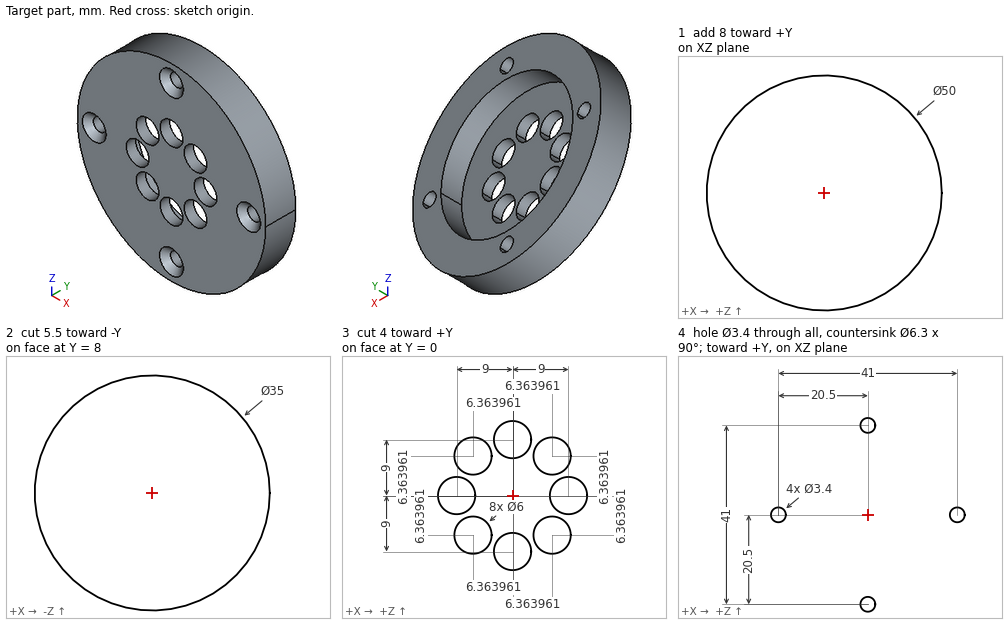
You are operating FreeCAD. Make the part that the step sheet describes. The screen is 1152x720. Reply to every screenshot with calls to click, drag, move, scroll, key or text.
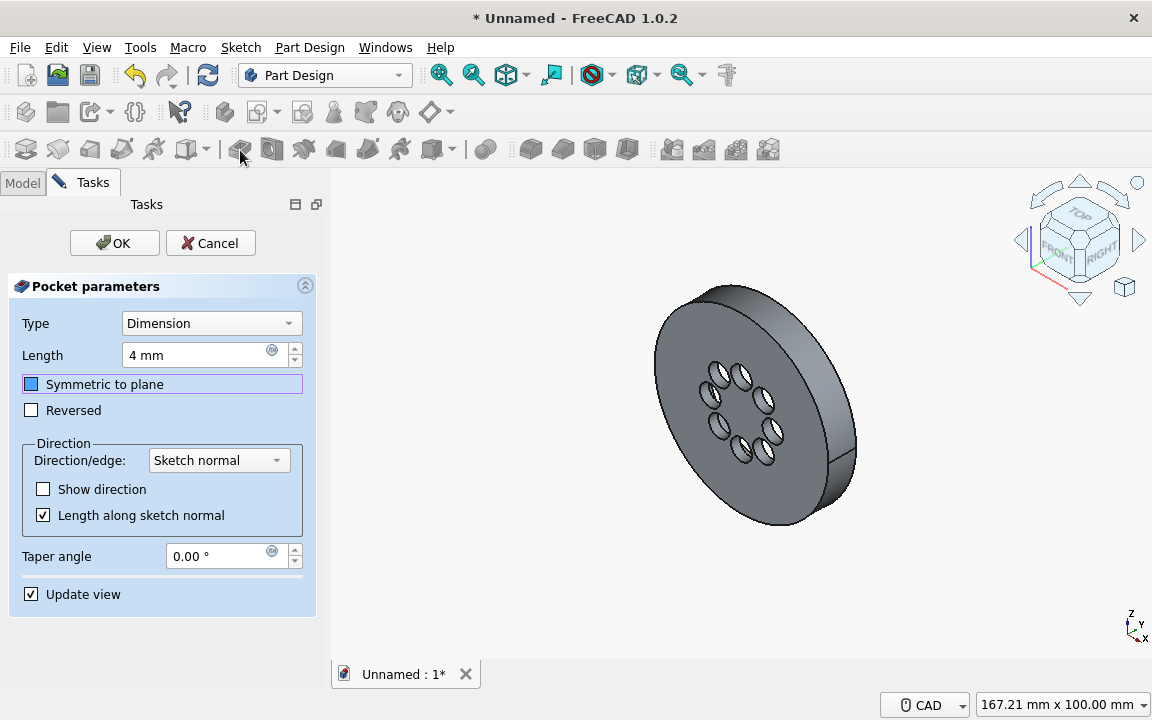
click(115, 243)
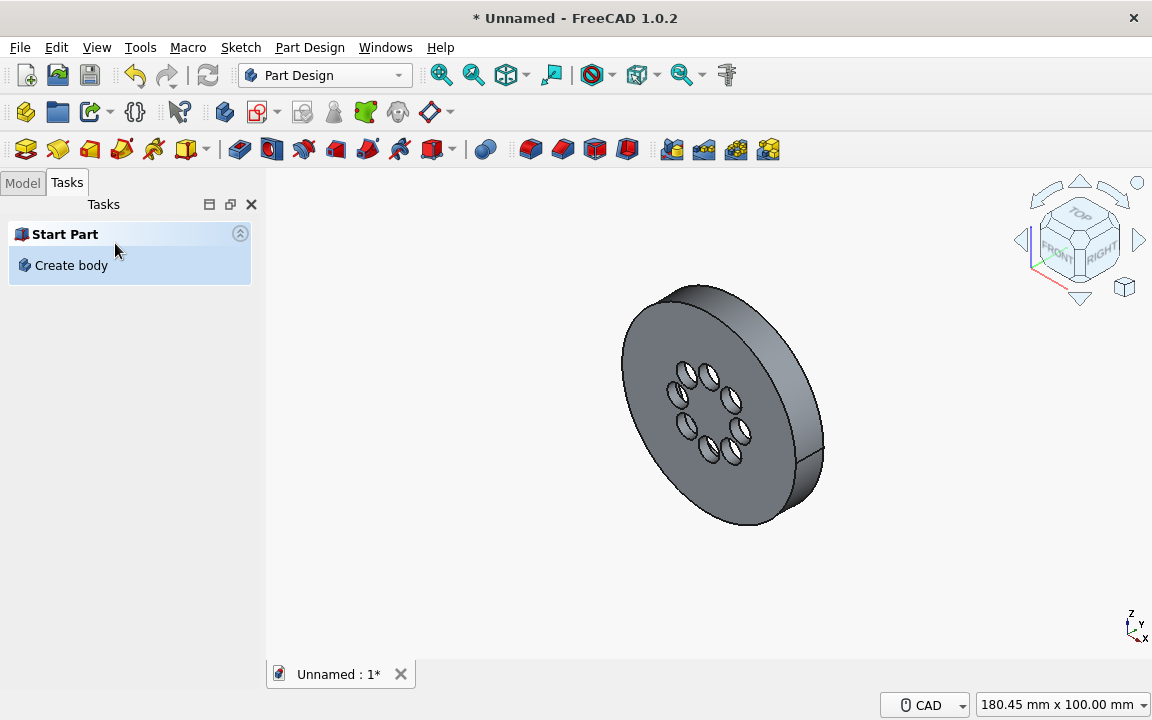
click(258, 112)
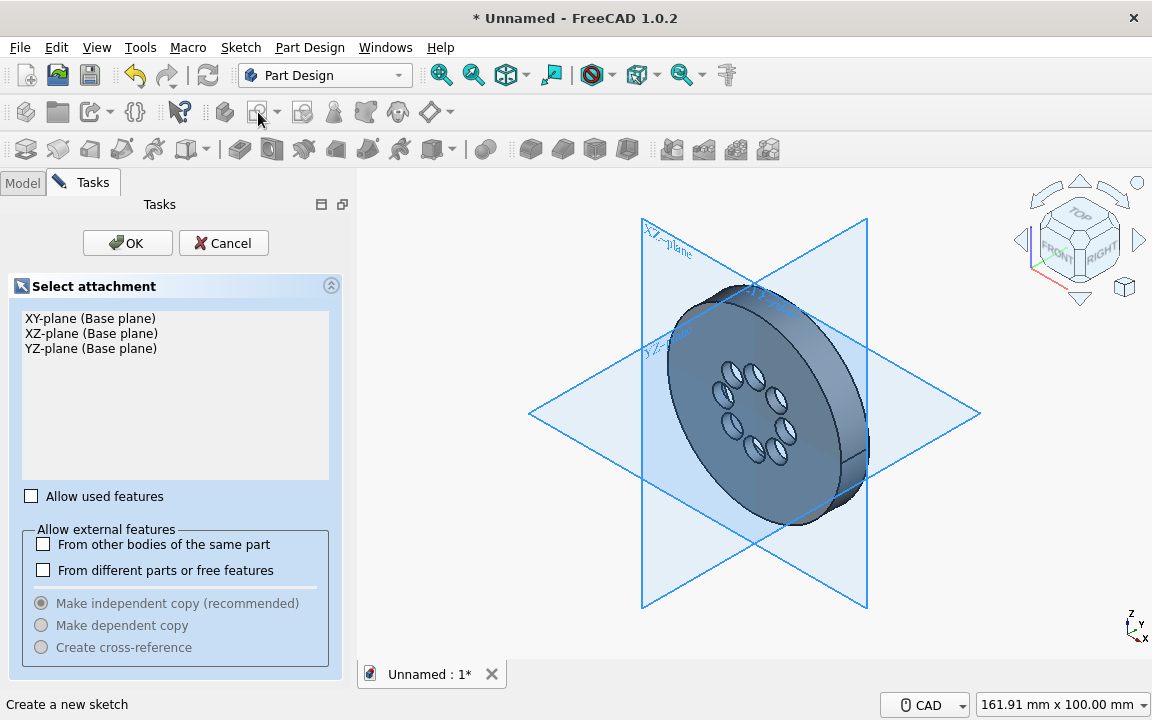
click(82, 334)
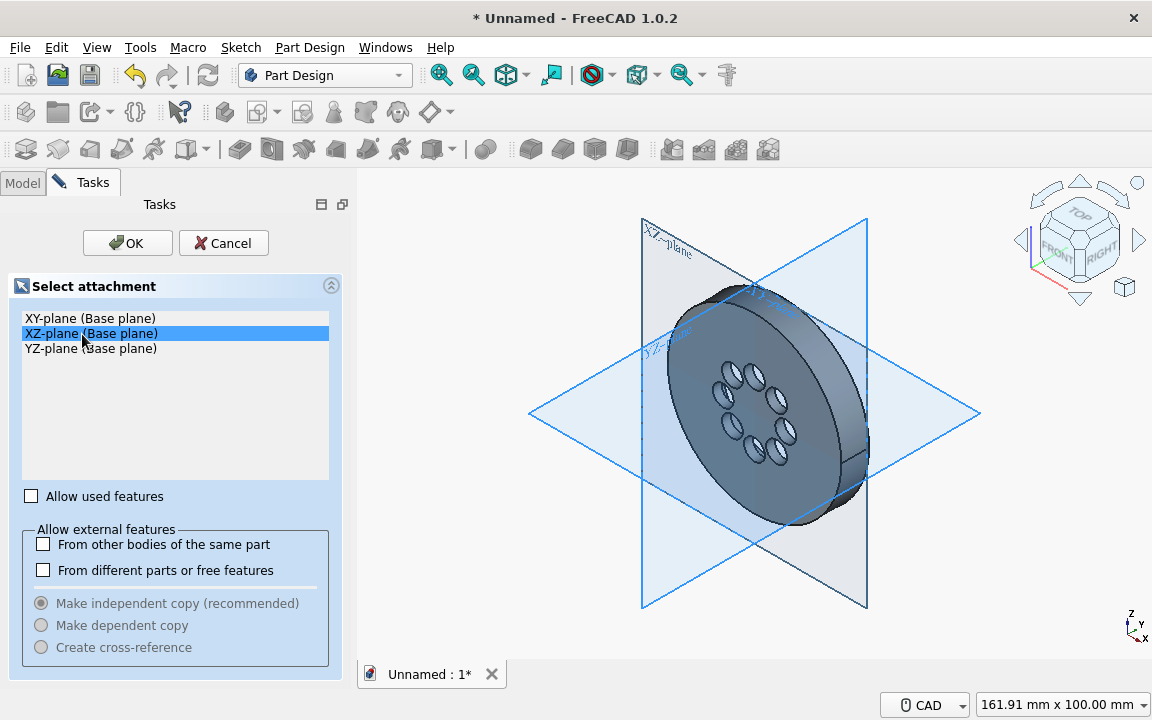
click(128, 243)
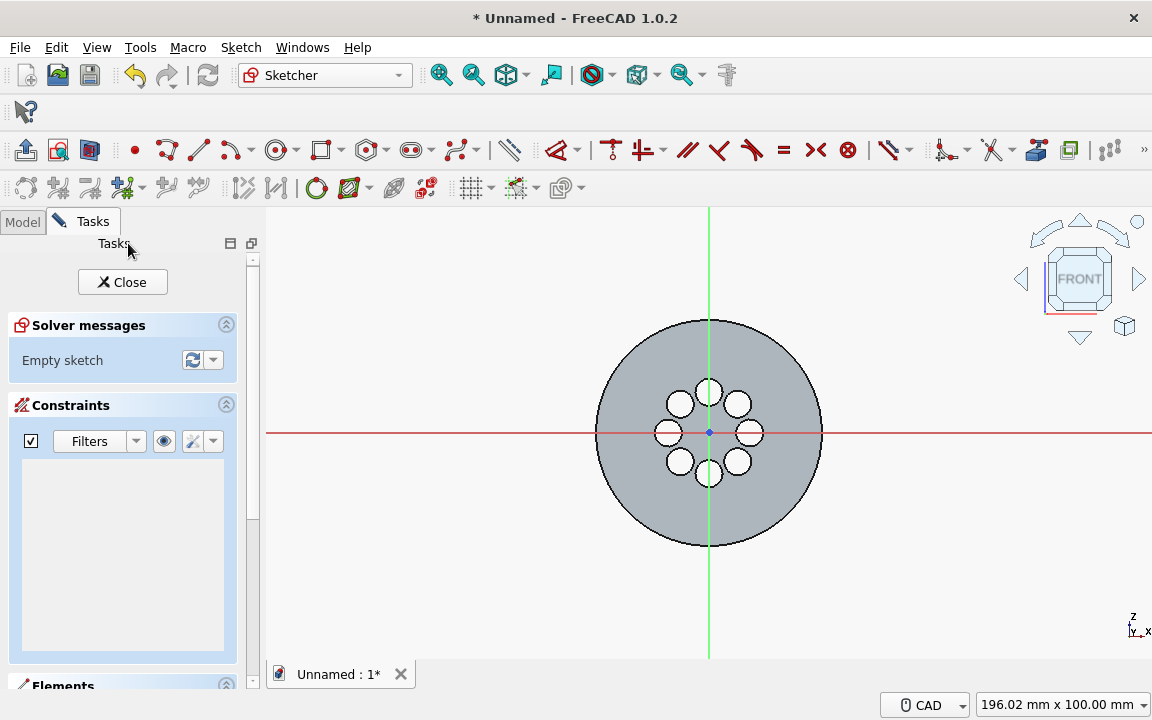
scroll(848, 433, up, 2)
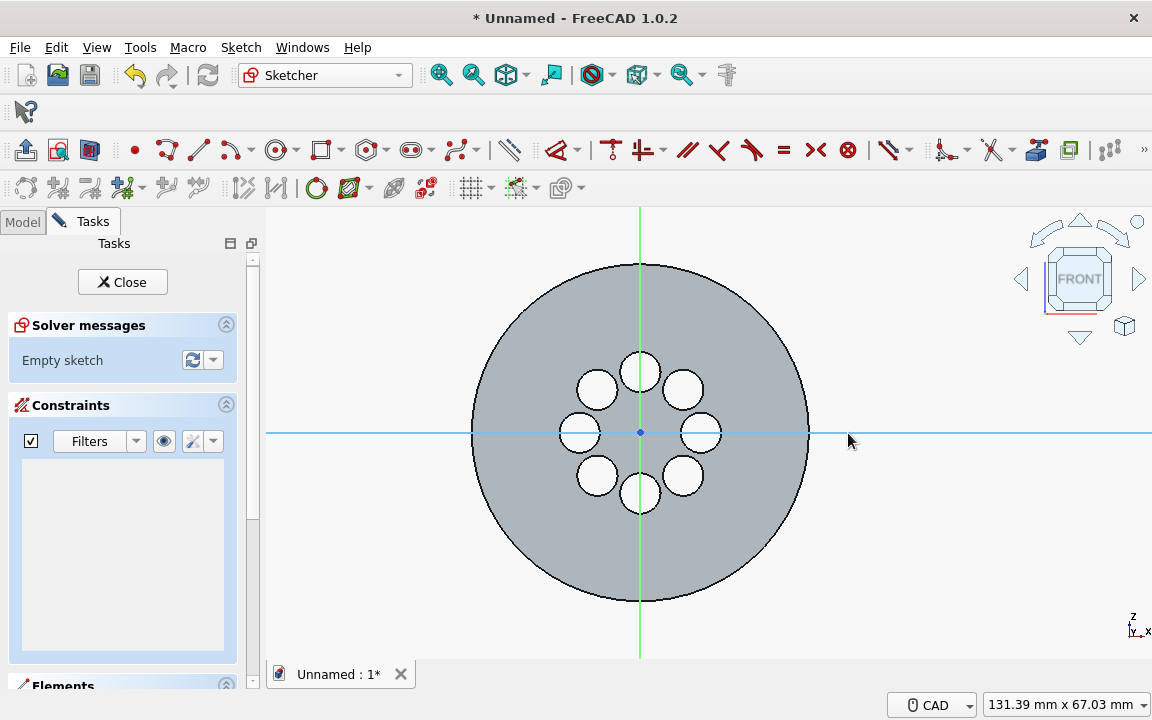
key(g)
key(c)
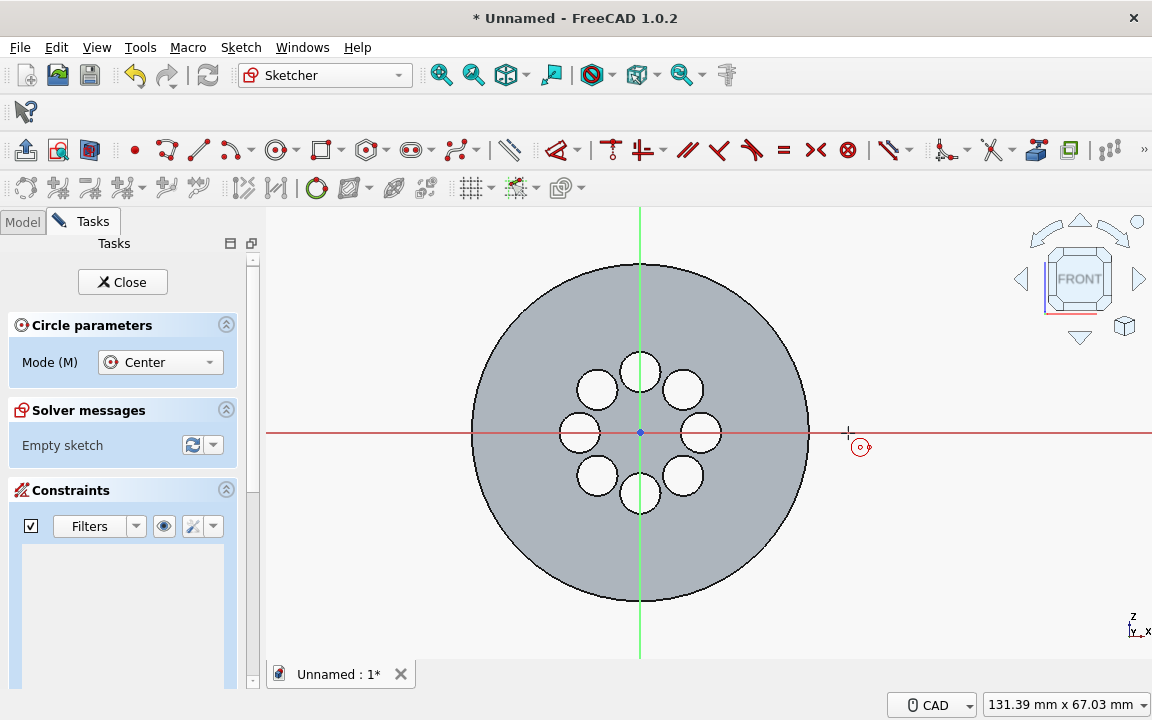
scroll(502, 433, up, 4)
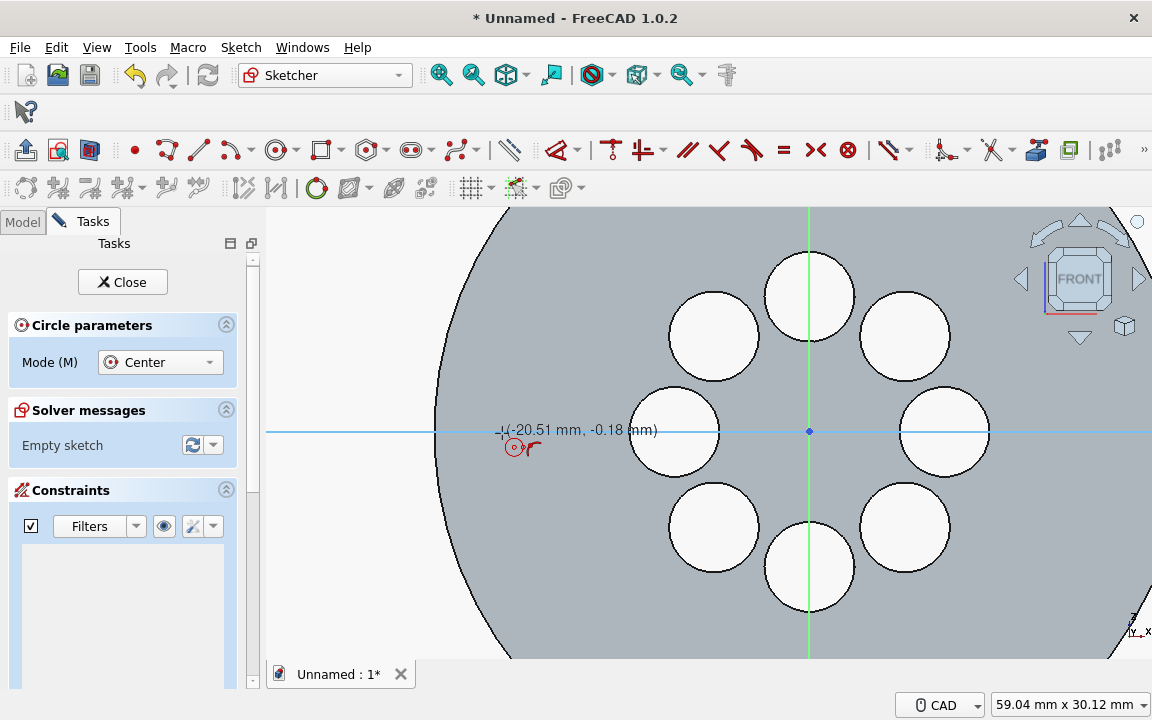
click(502, 432)
move(520, 414)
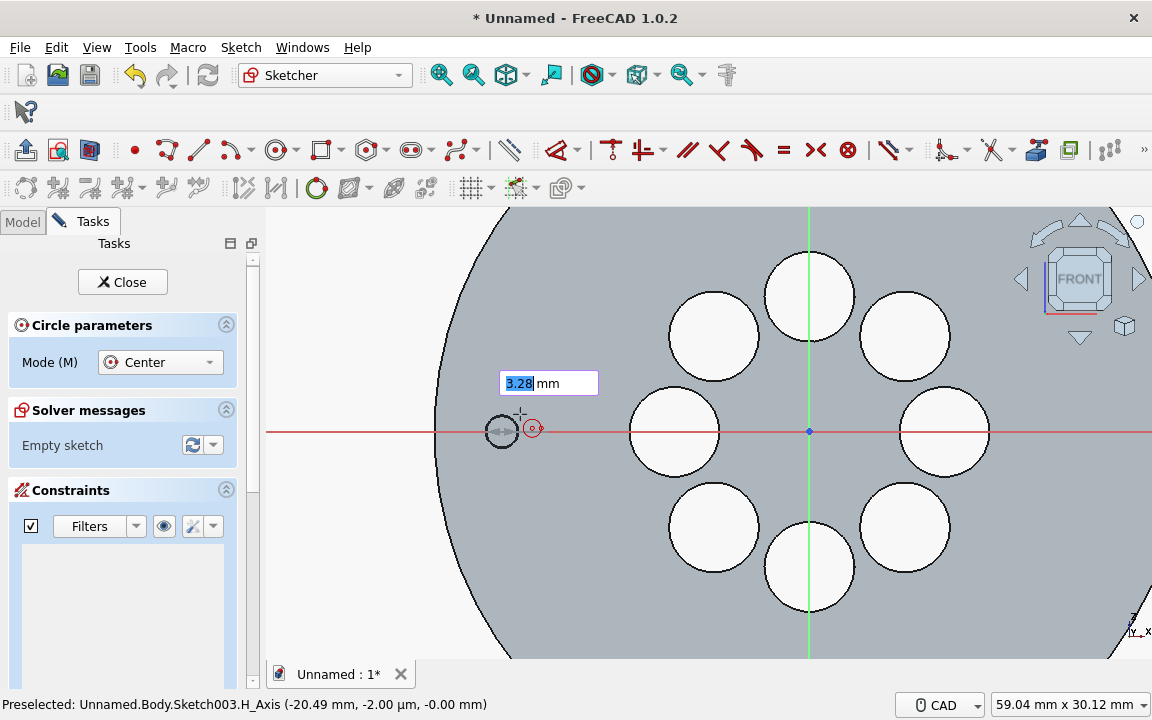
text(3.4)
key(Return)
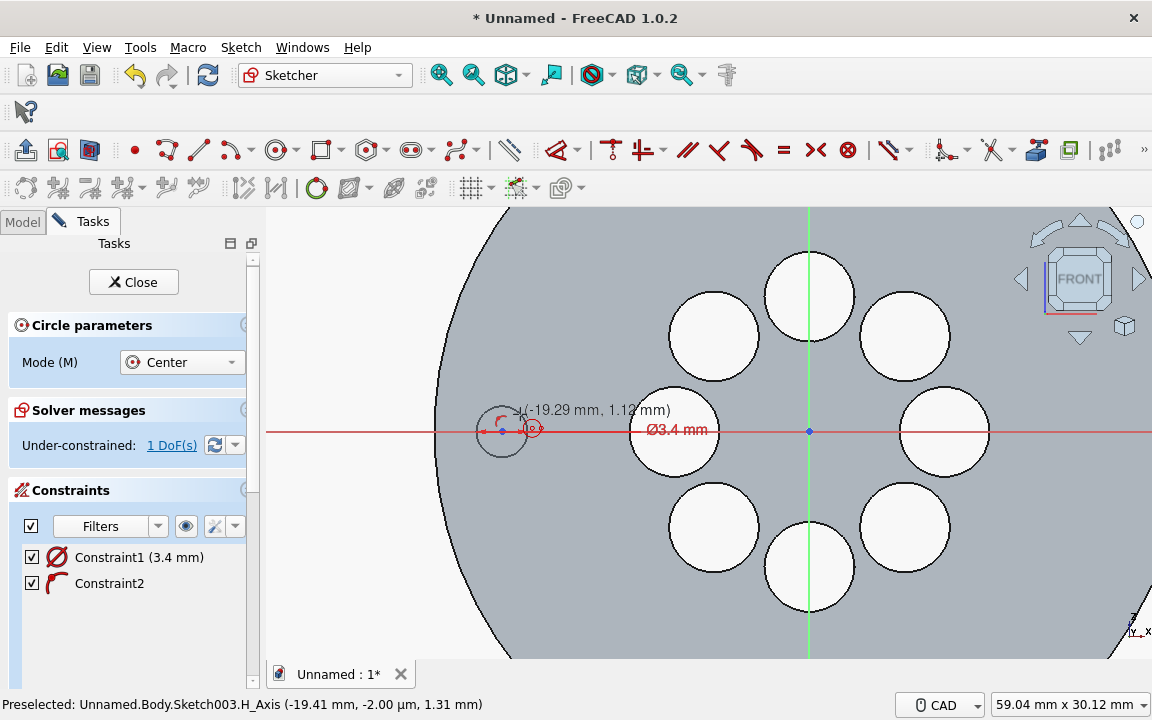
scroll(503, 434, down, 4)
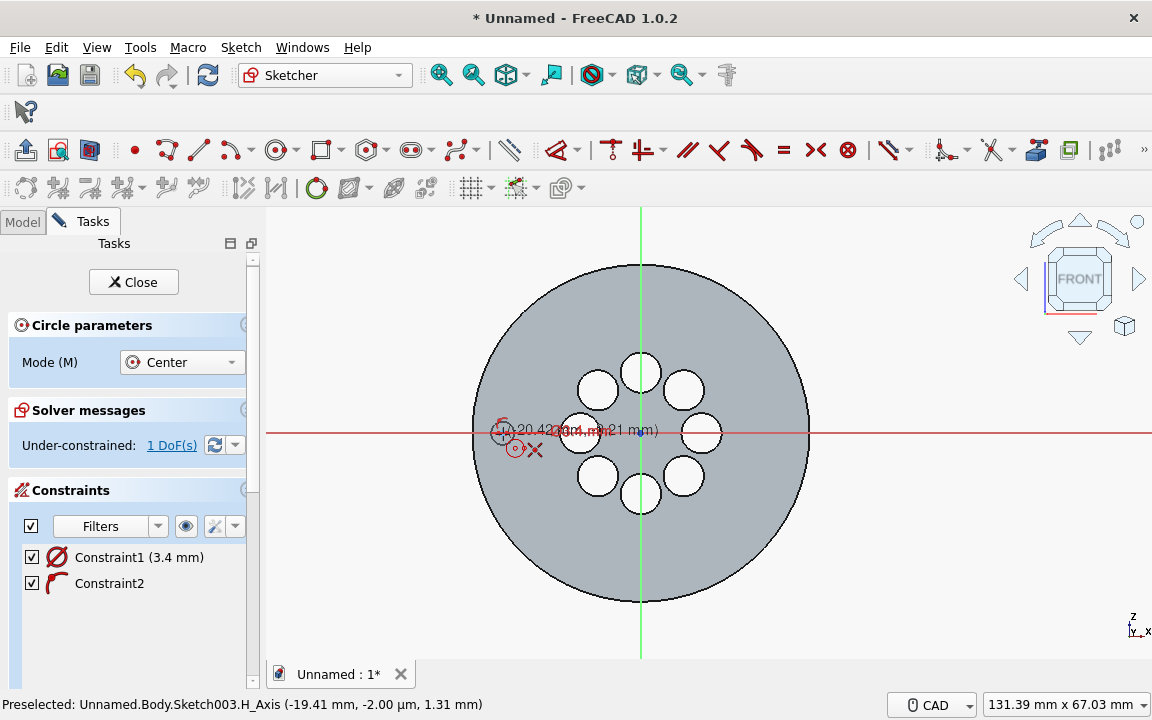
scroll(641, 572, up, 4)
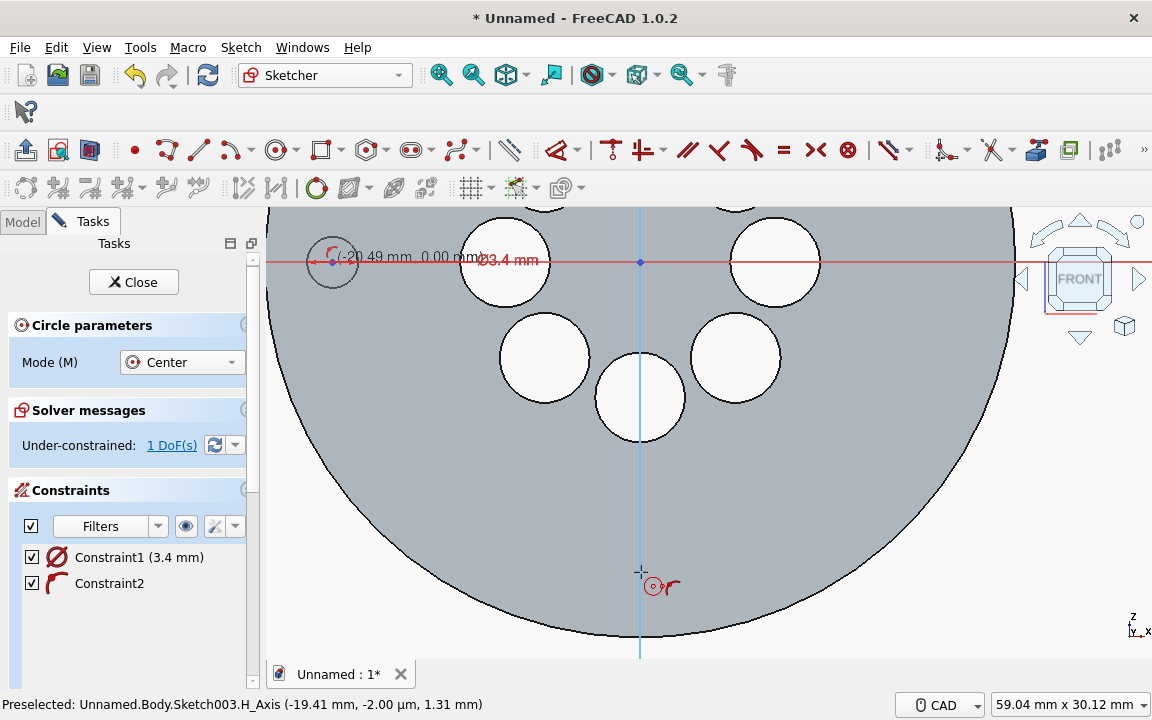
click(640, 570)
move(658, 552)